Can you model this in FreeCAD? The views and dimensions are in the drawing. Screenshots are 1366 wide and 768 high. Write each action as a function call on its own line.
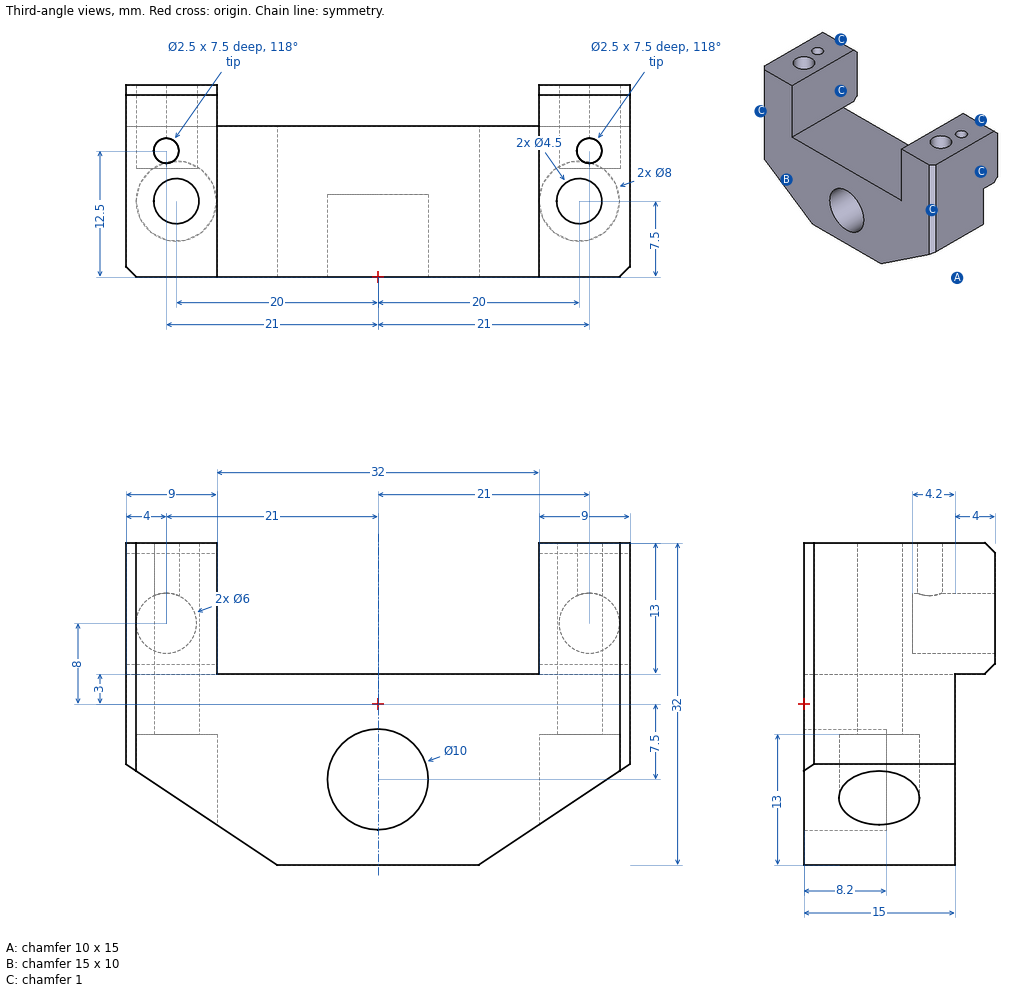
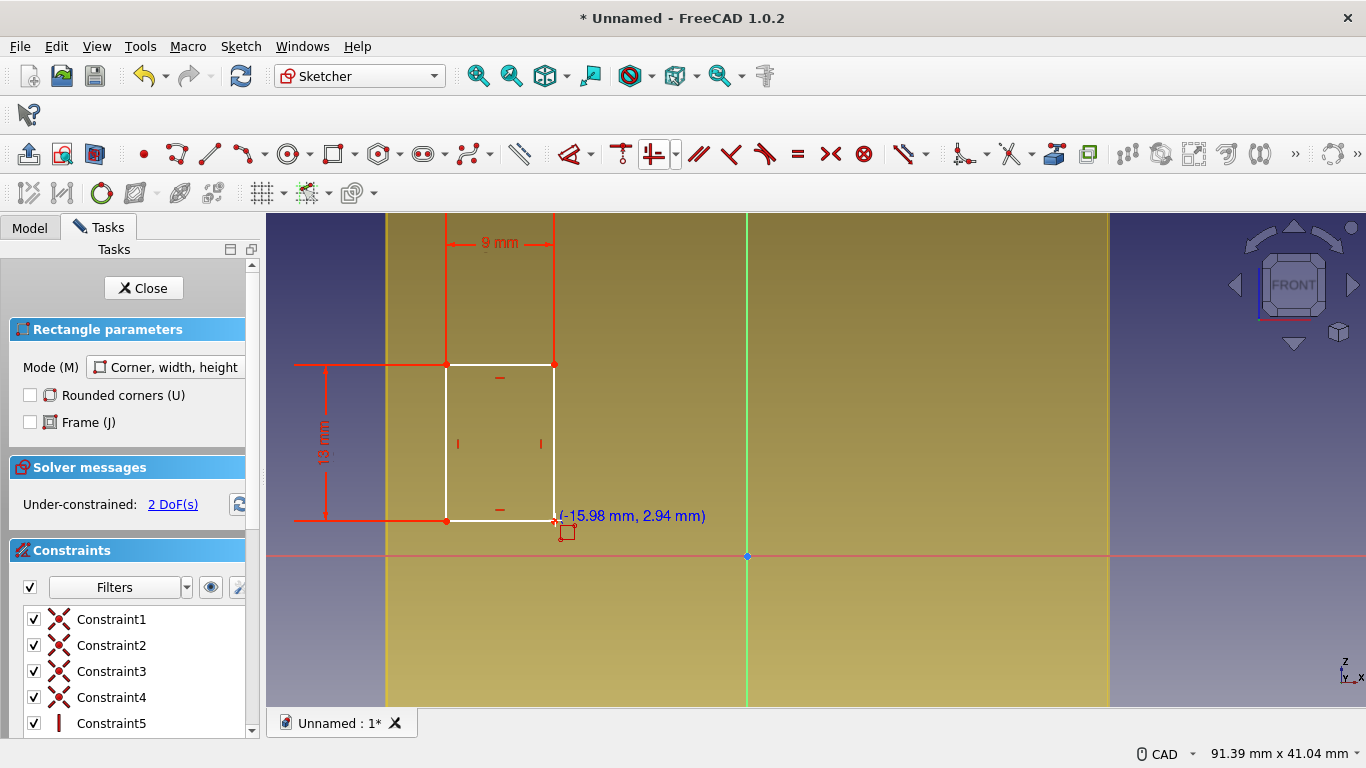
click(940, 364)
move(1048, 520)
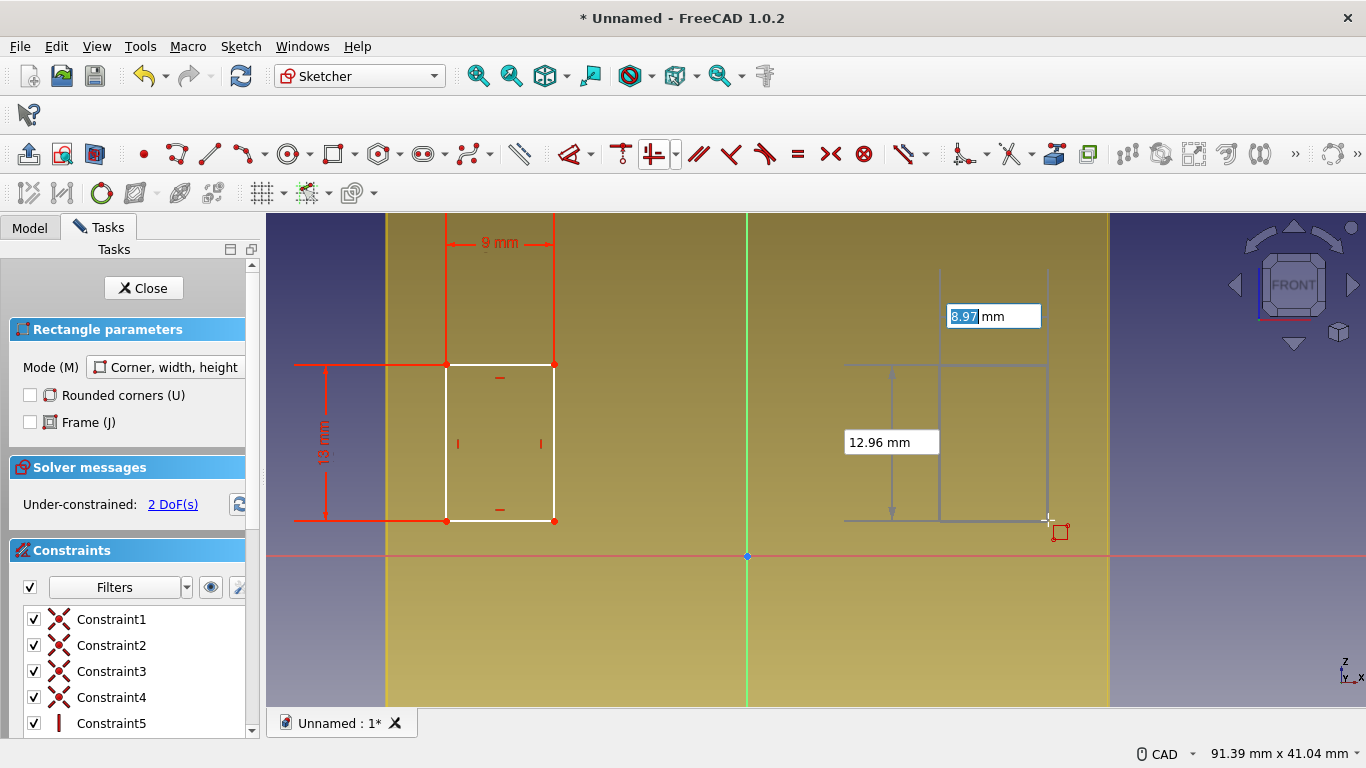
text(9)
key(Tab)
text(13)
key(Return)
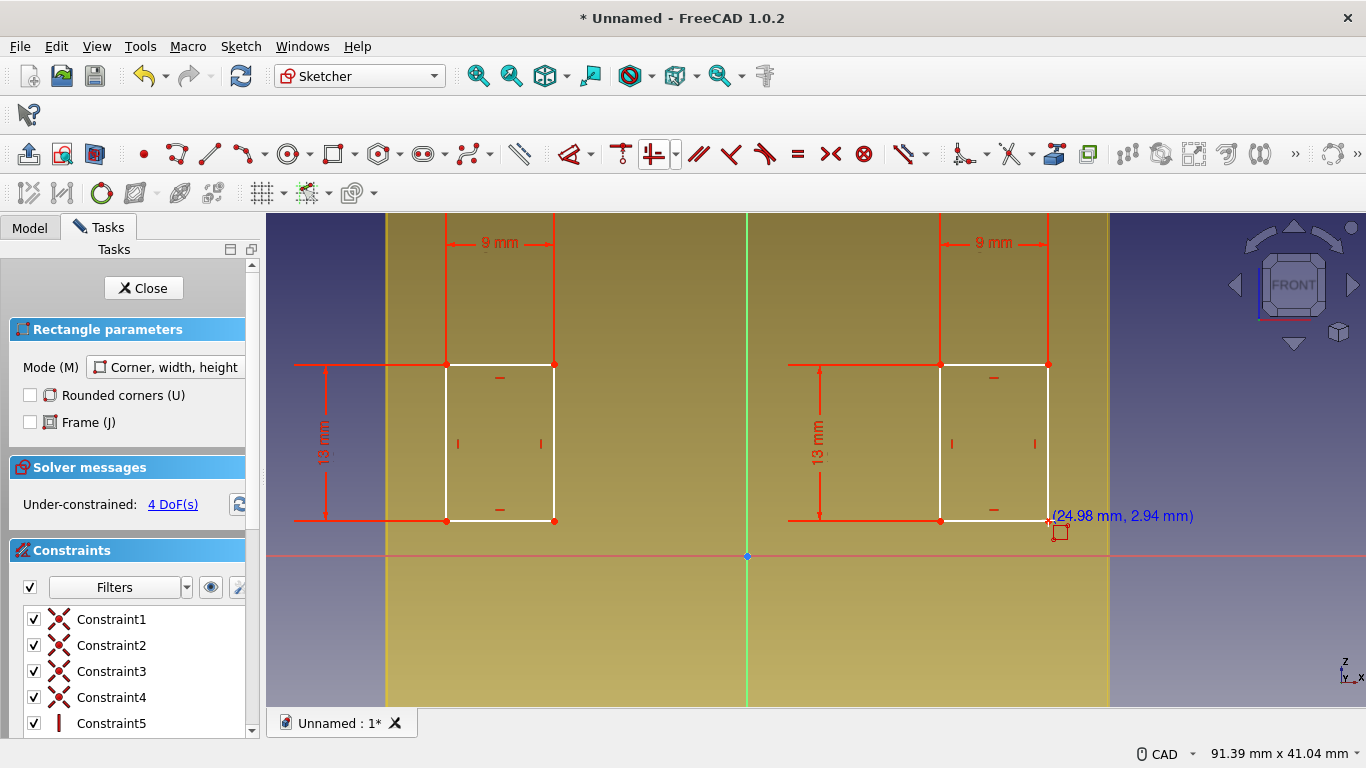
click(288, 154)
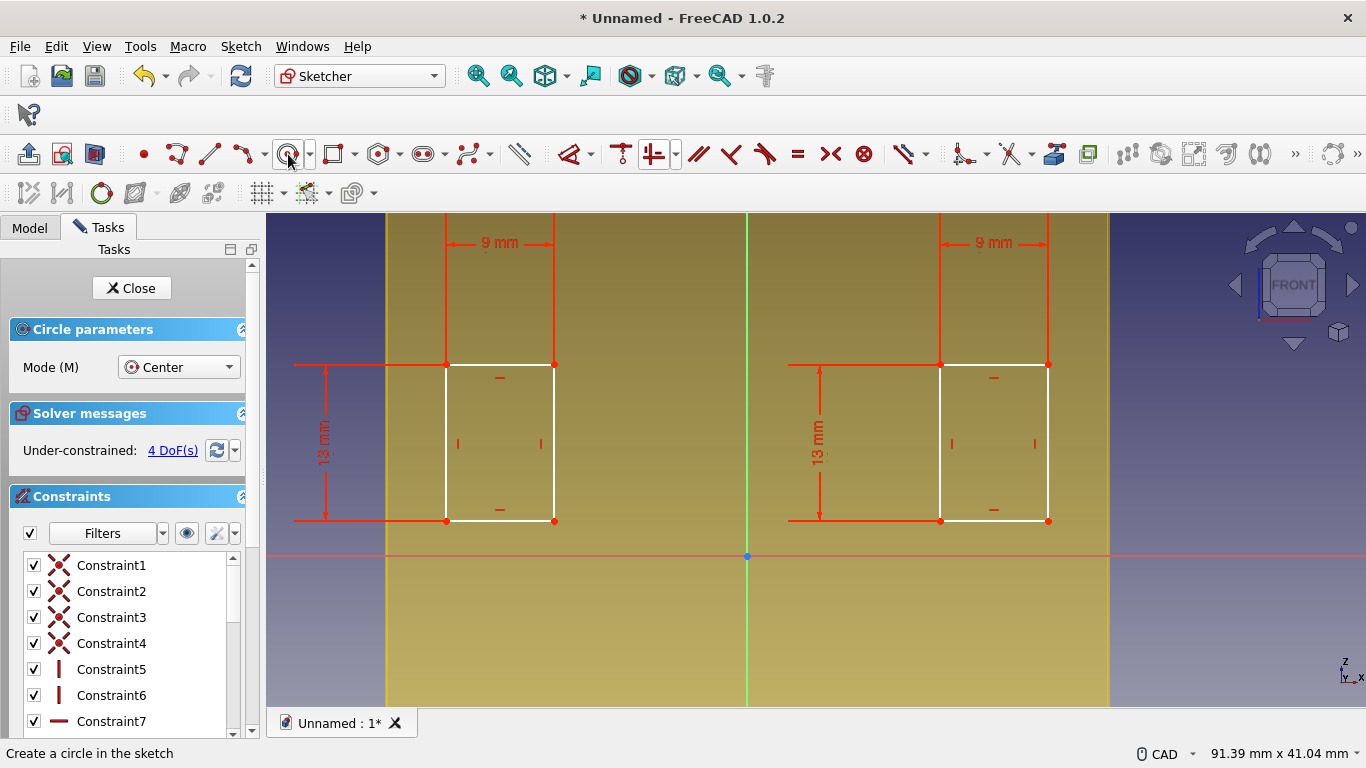
click(495, 460)
move(520, 435)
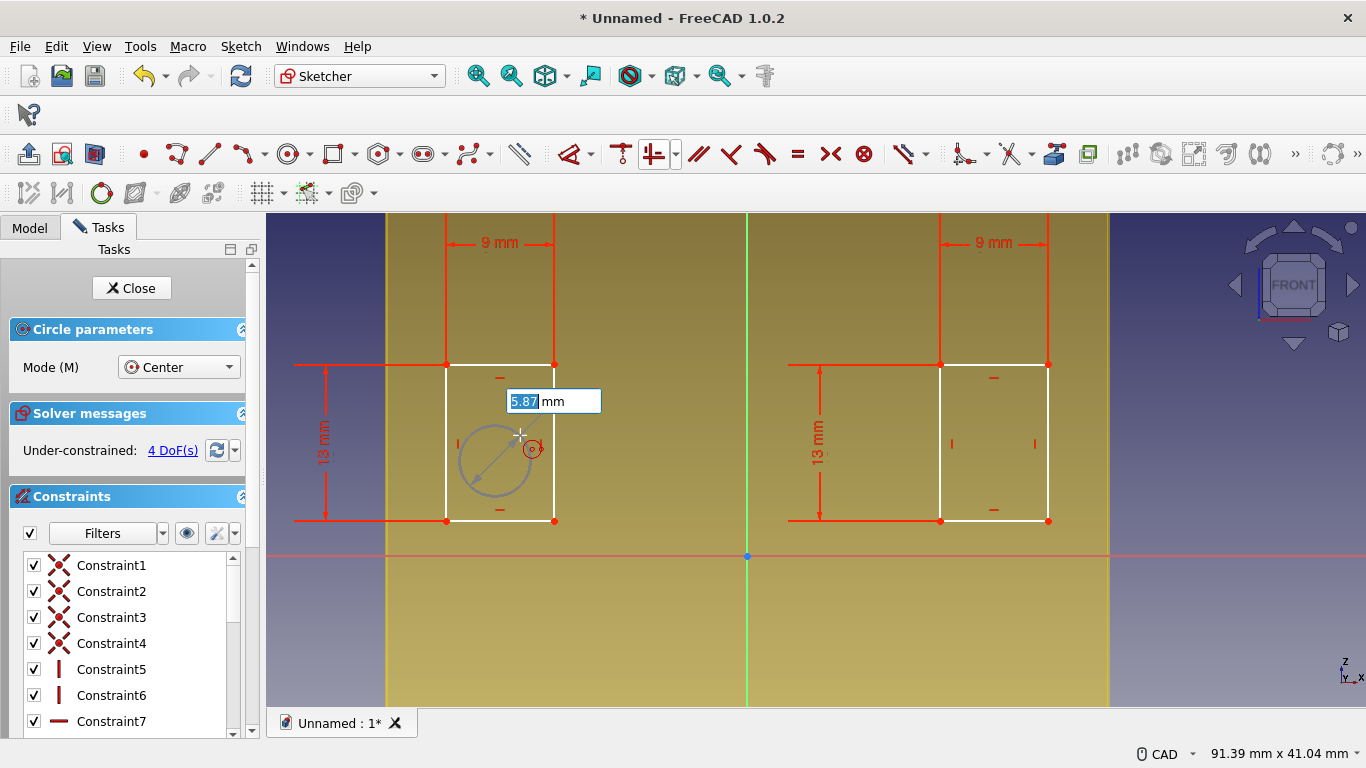
text(6)
key(Return)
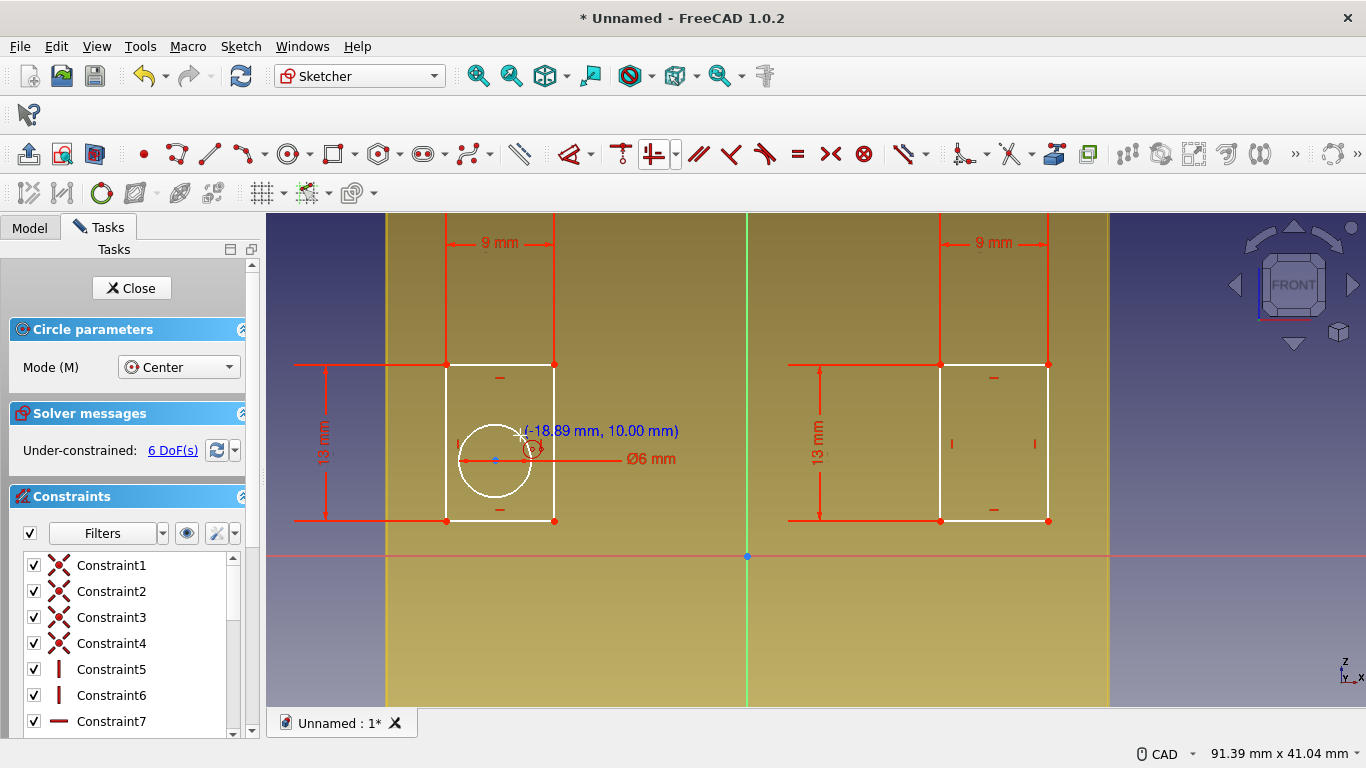
click(1000, 460)
move(1026, 435)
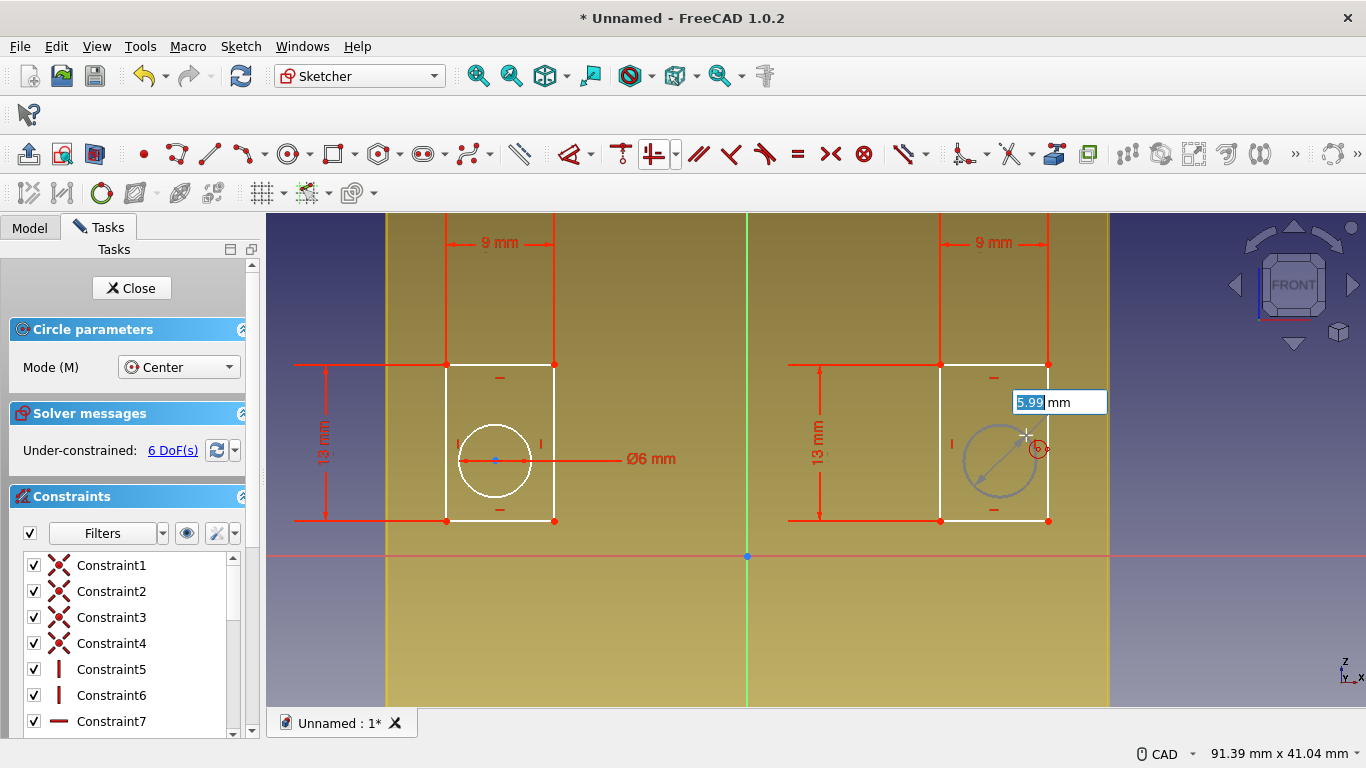
text(6)
key(Return)
key(Escape)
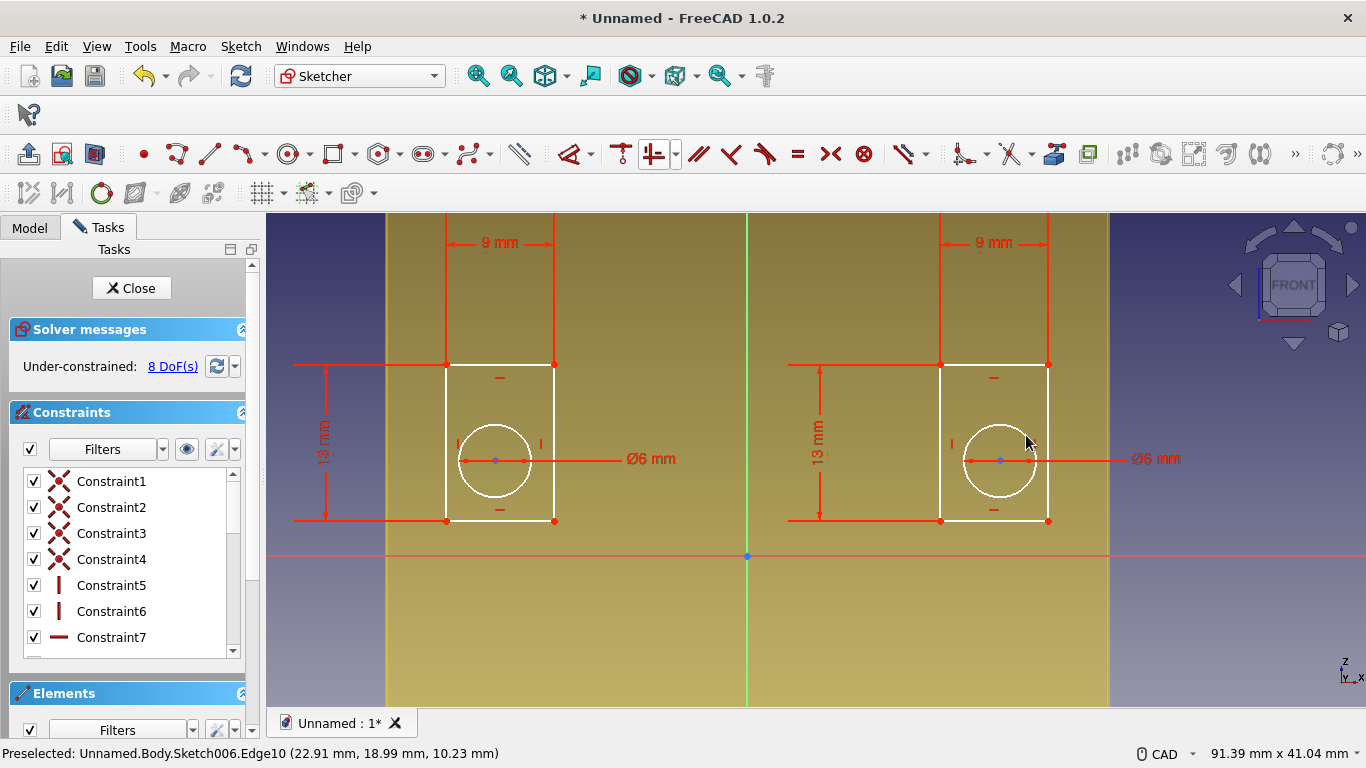
click(495, 461)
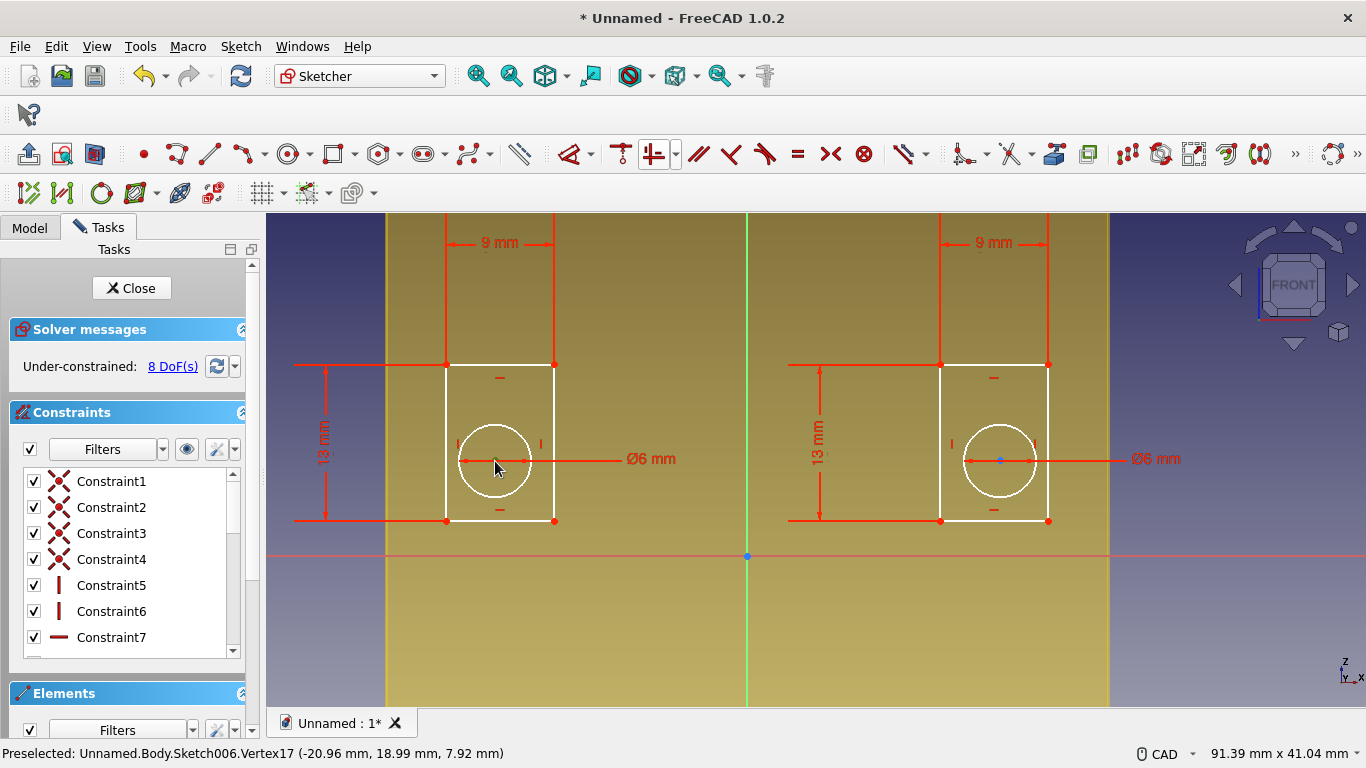
click(1000, 461)